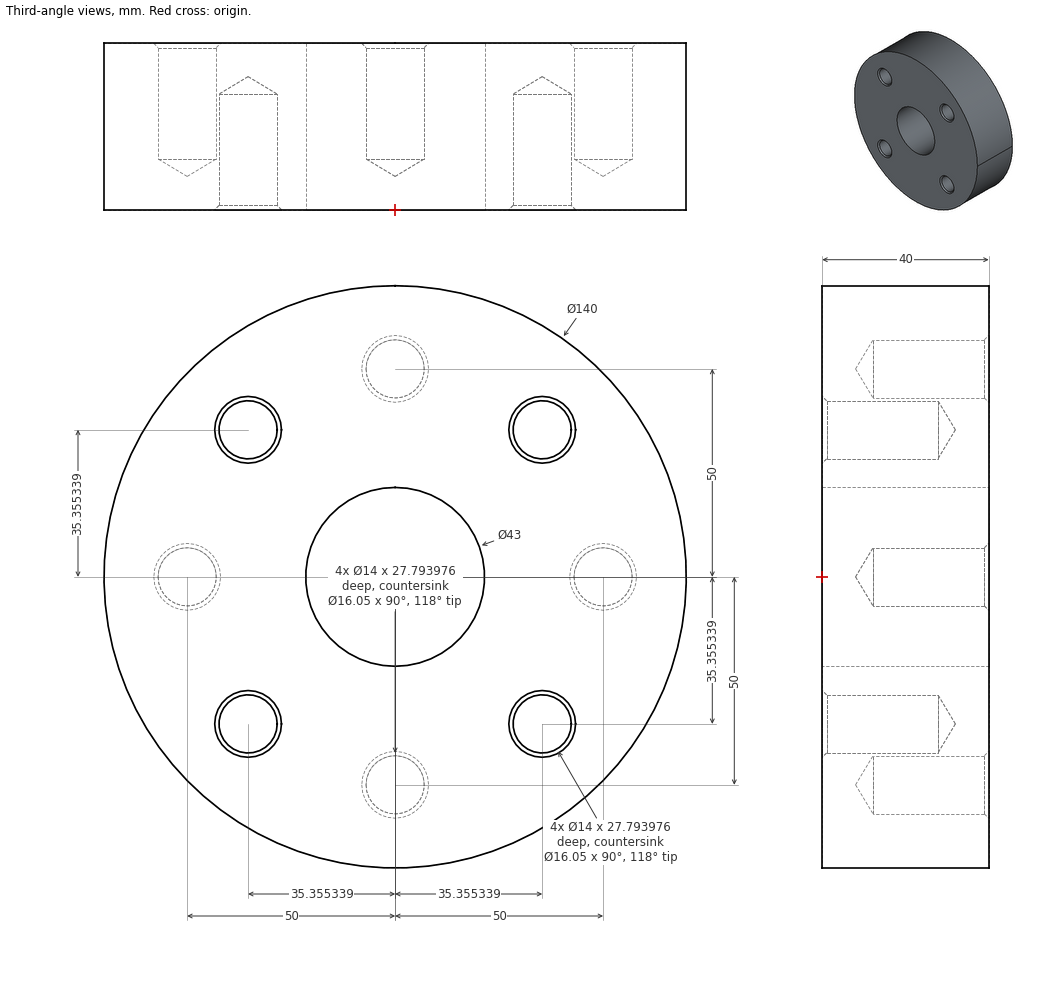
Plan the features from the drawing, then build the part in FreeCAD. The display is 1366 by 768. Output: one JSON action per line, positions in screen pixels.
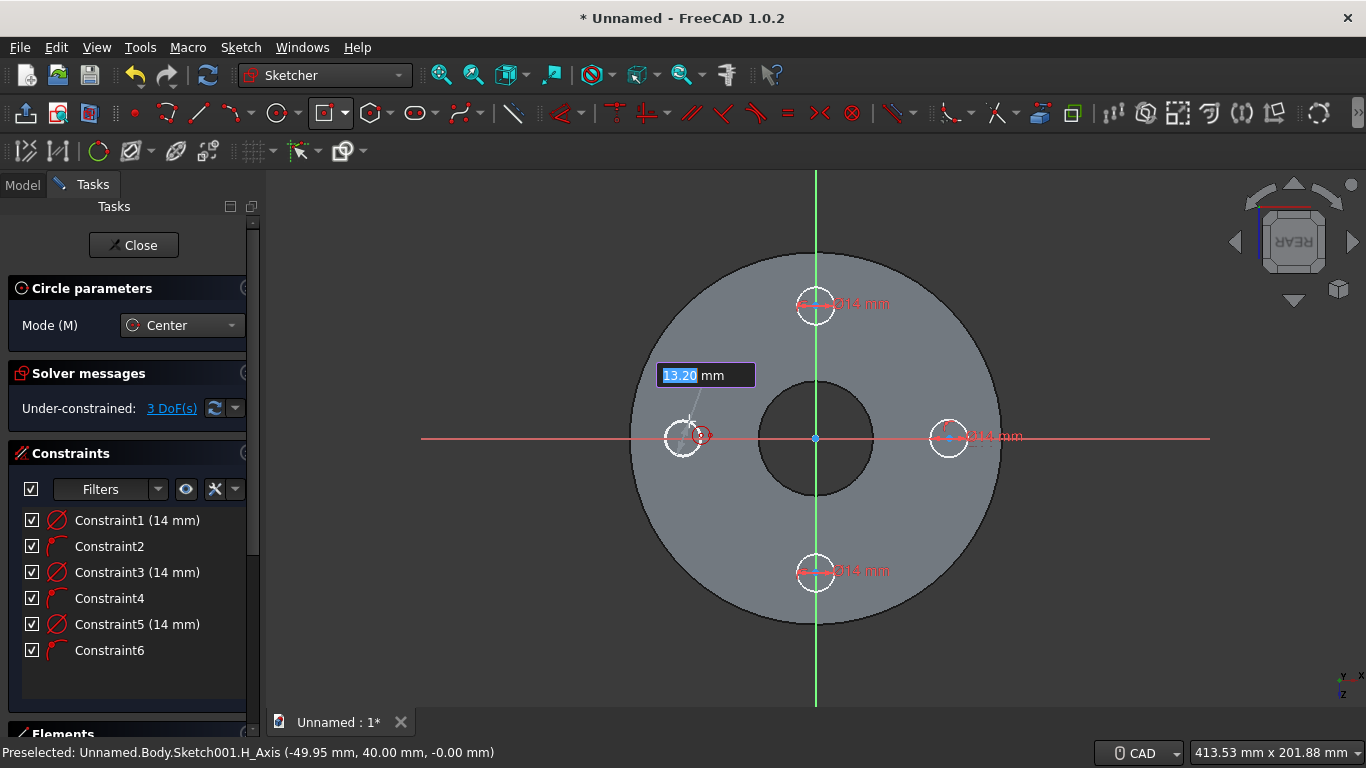
{"action": "type", "text": "14"}
{"action": "key", "text": "Return"}
{"action": "key", "text": "Escape"}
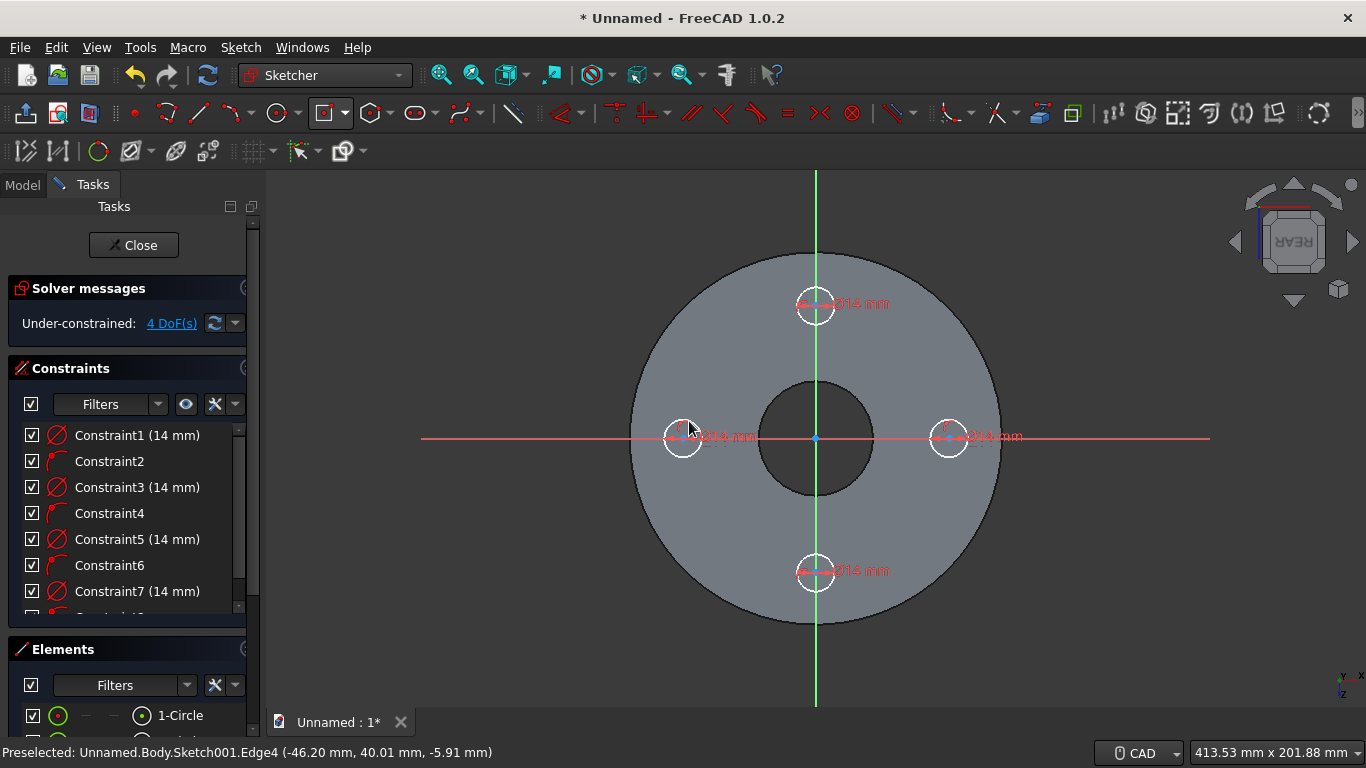
{"action": "left_click", "coordinate": [816, 306]}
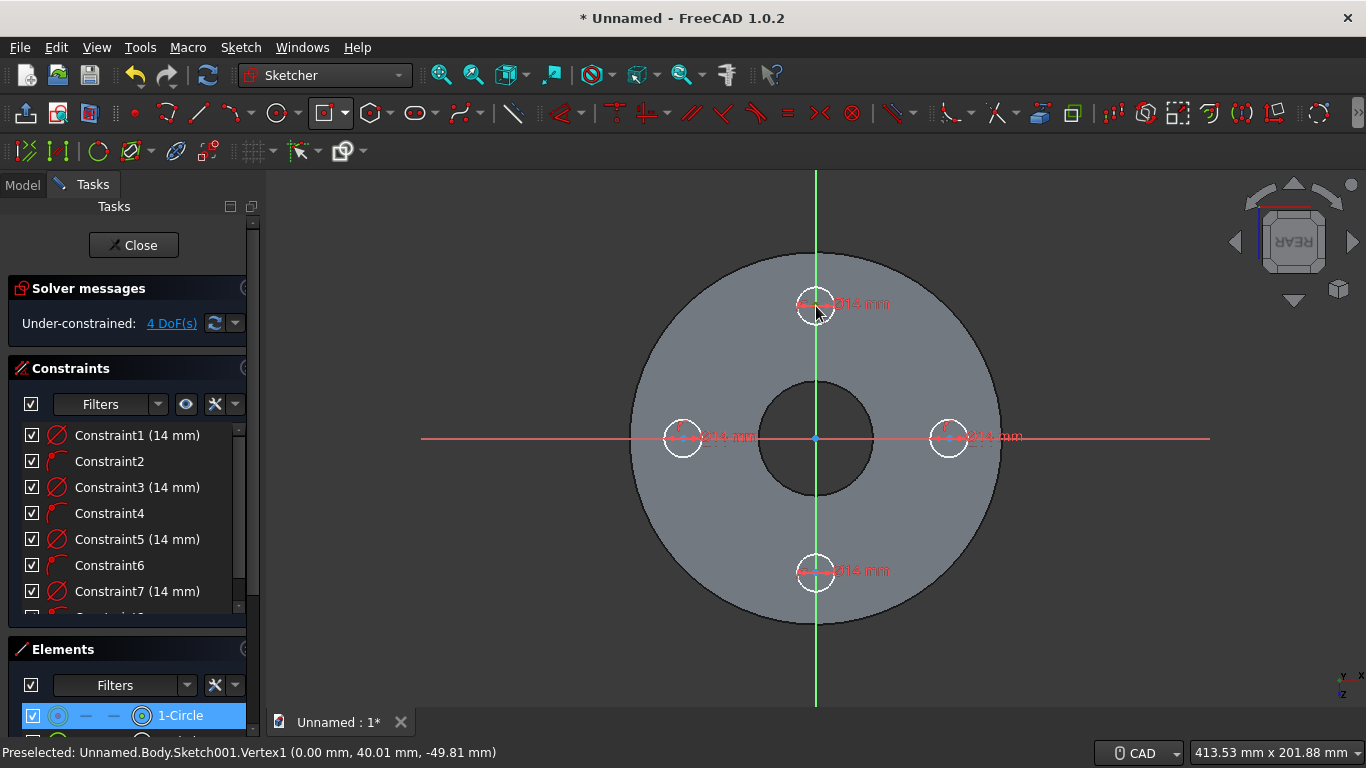
{"action": "key", "text": "i"}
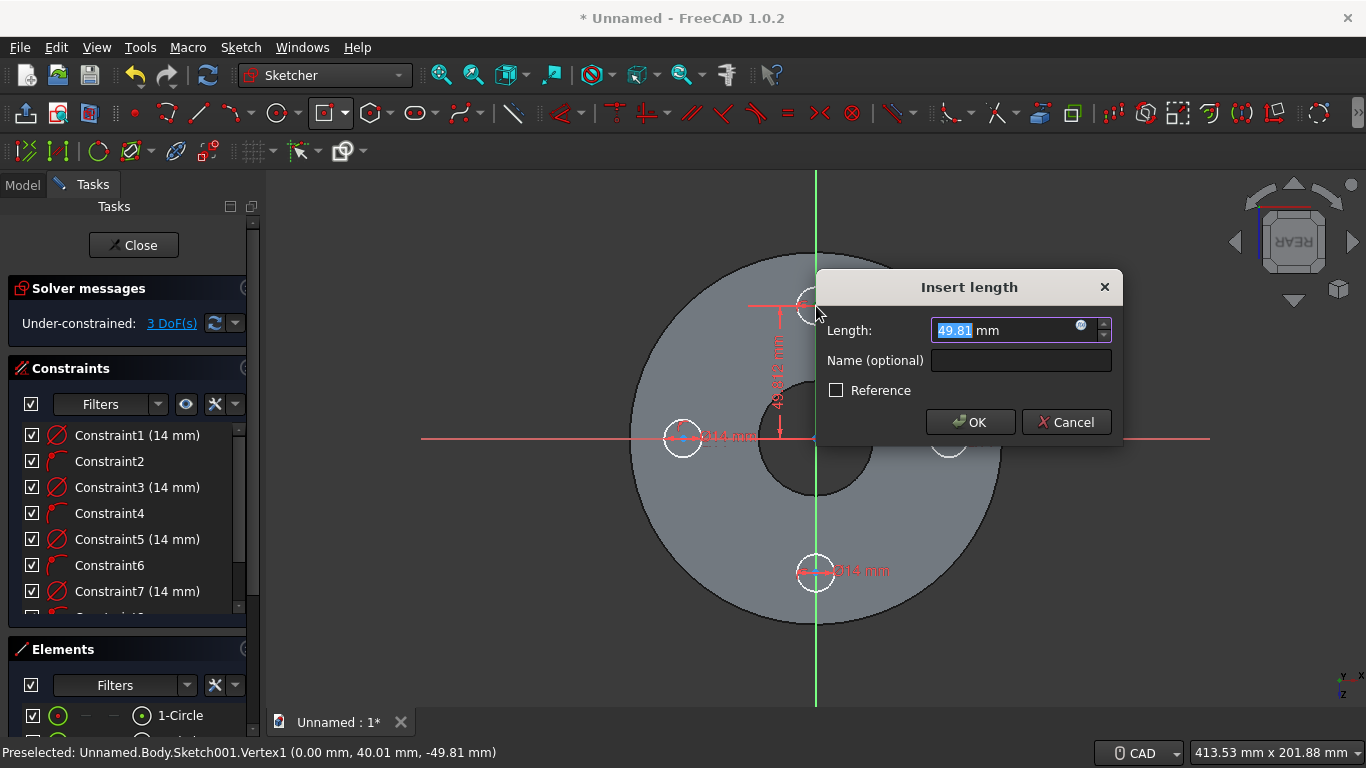
{"action": "type", "text": "50"}
{"action": "key", "text": "Return"}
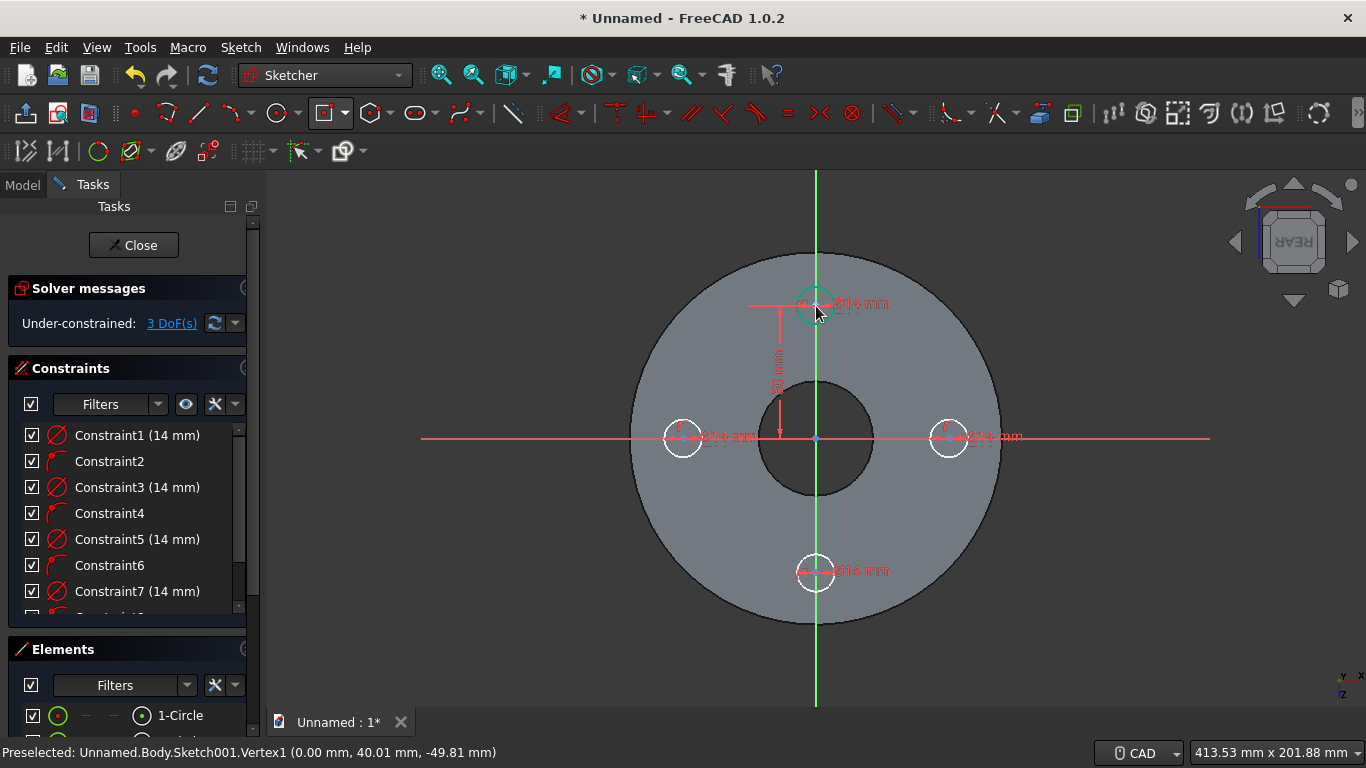
{"action": "left_click", "coordinate": [949, 439]}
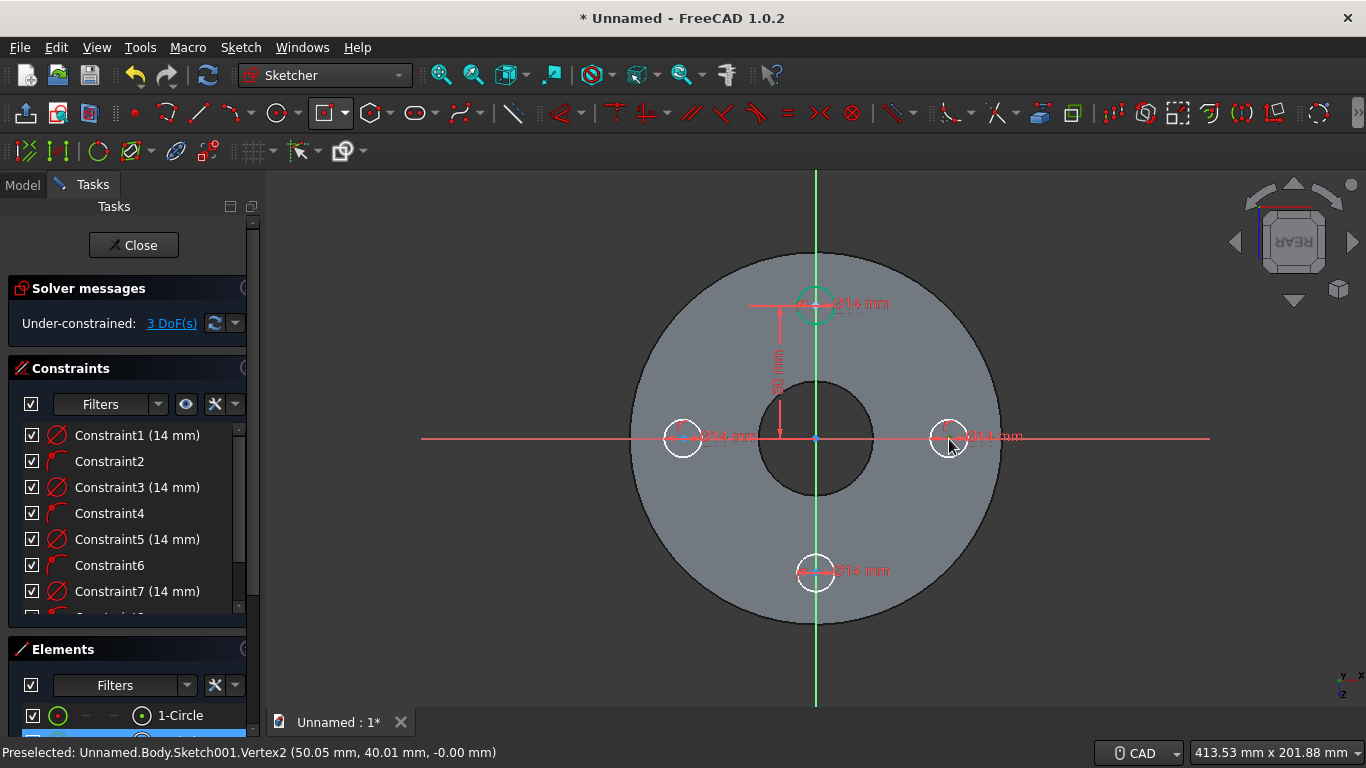
{"action": "left_click", "coordinate": [584, 114]}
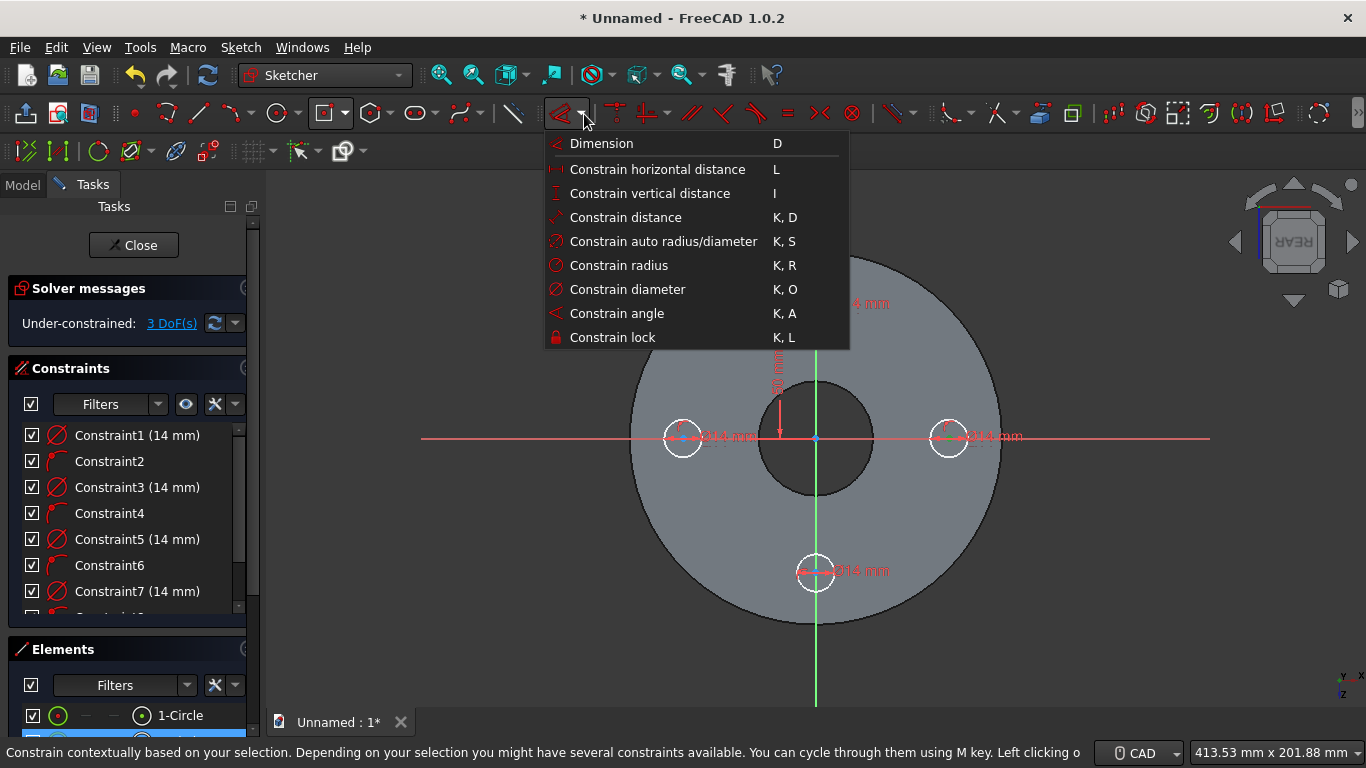
{"action": "left_click", "coordinate": [697, 169]}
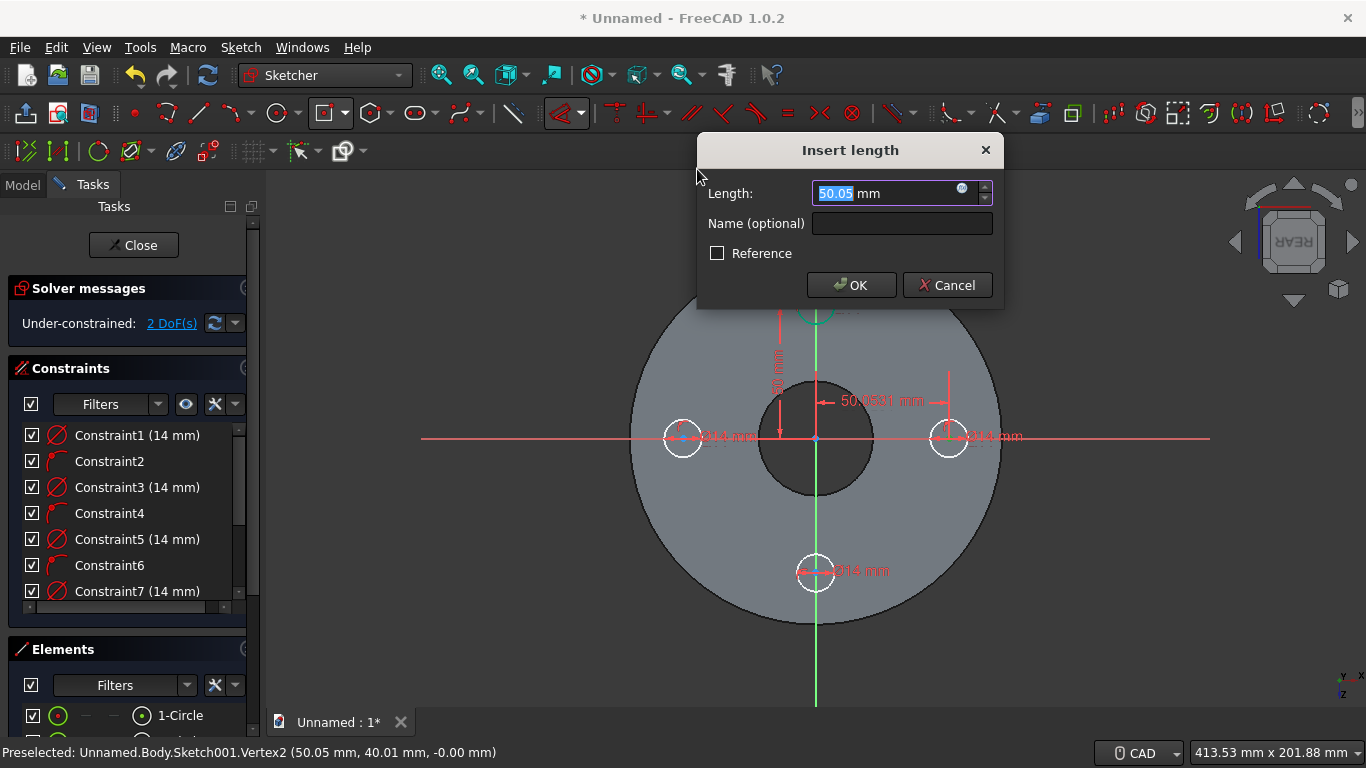
{"action": "type", "text": "50"}
{"action": "key", "text": "Return"}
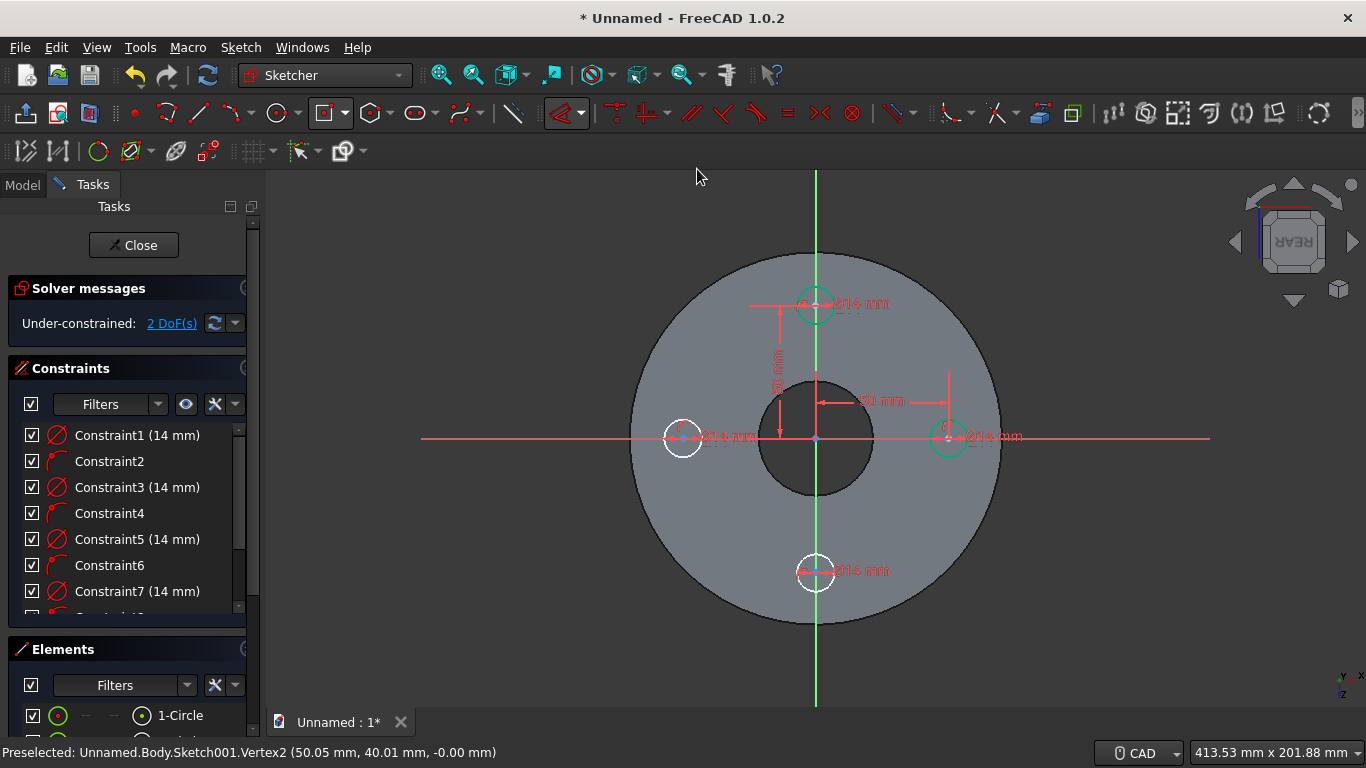
{"action": "left_click", "coordinate": [816, 573]}